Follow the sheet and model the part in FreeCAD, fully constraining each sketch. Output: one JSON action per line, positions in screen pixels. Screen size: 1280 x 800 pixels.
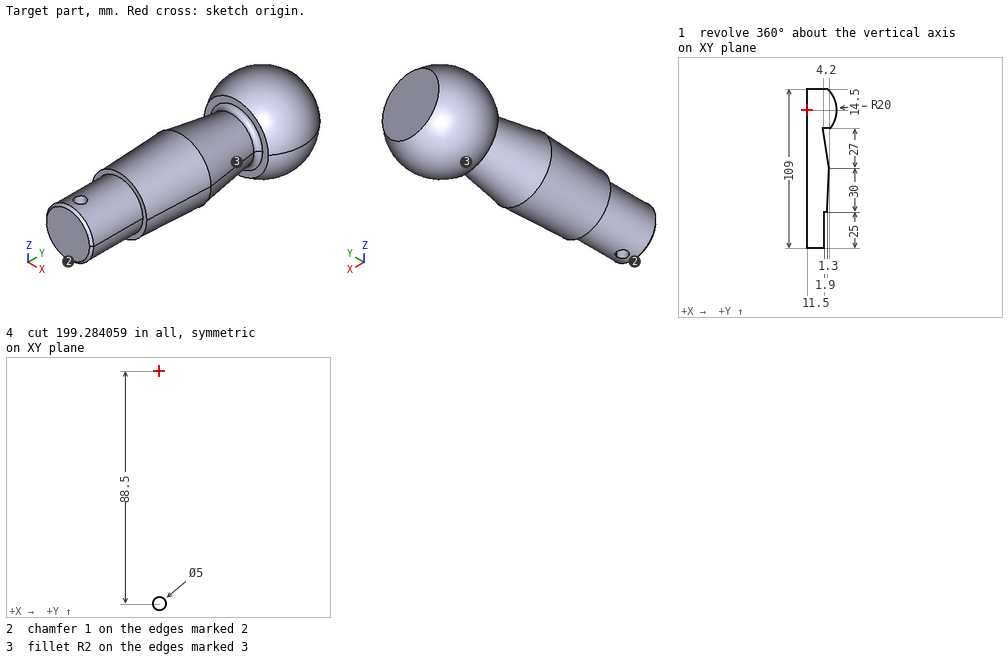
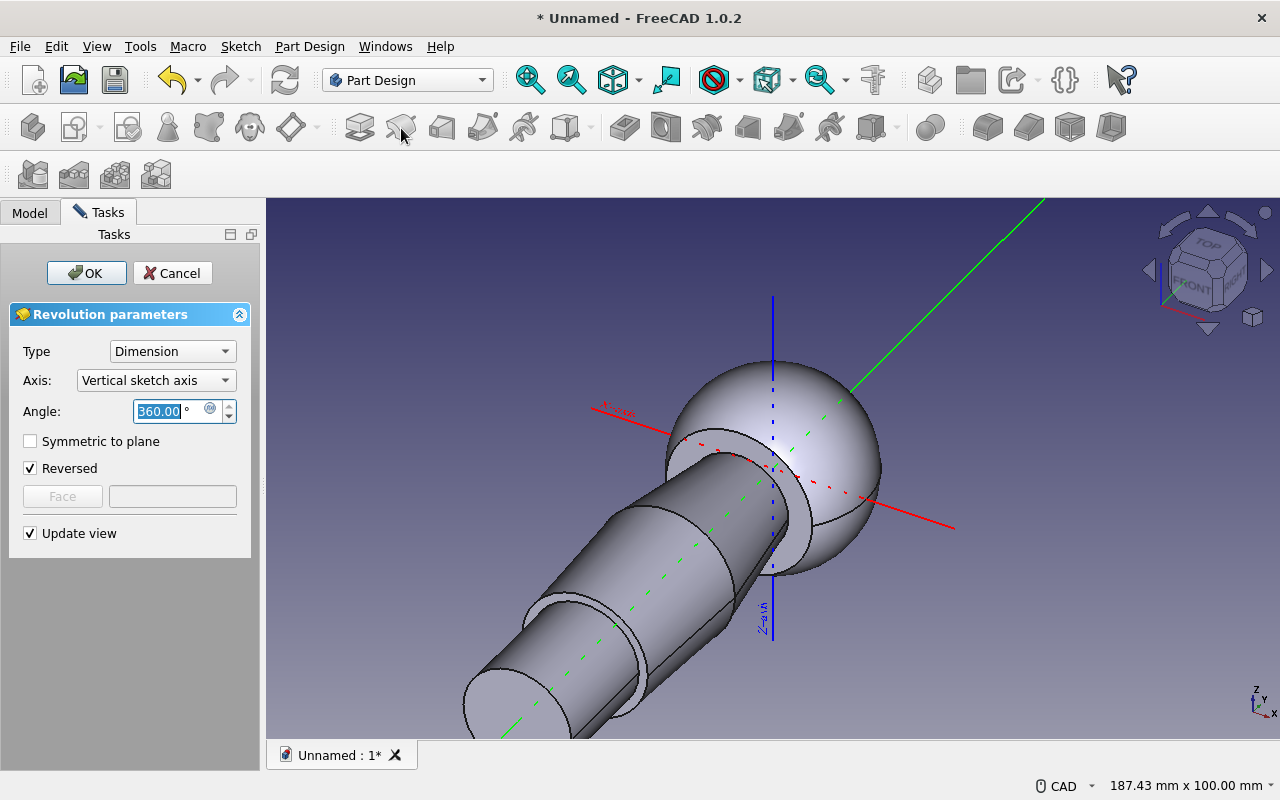
{"action": "left_click", "coordinate": [87, 273]}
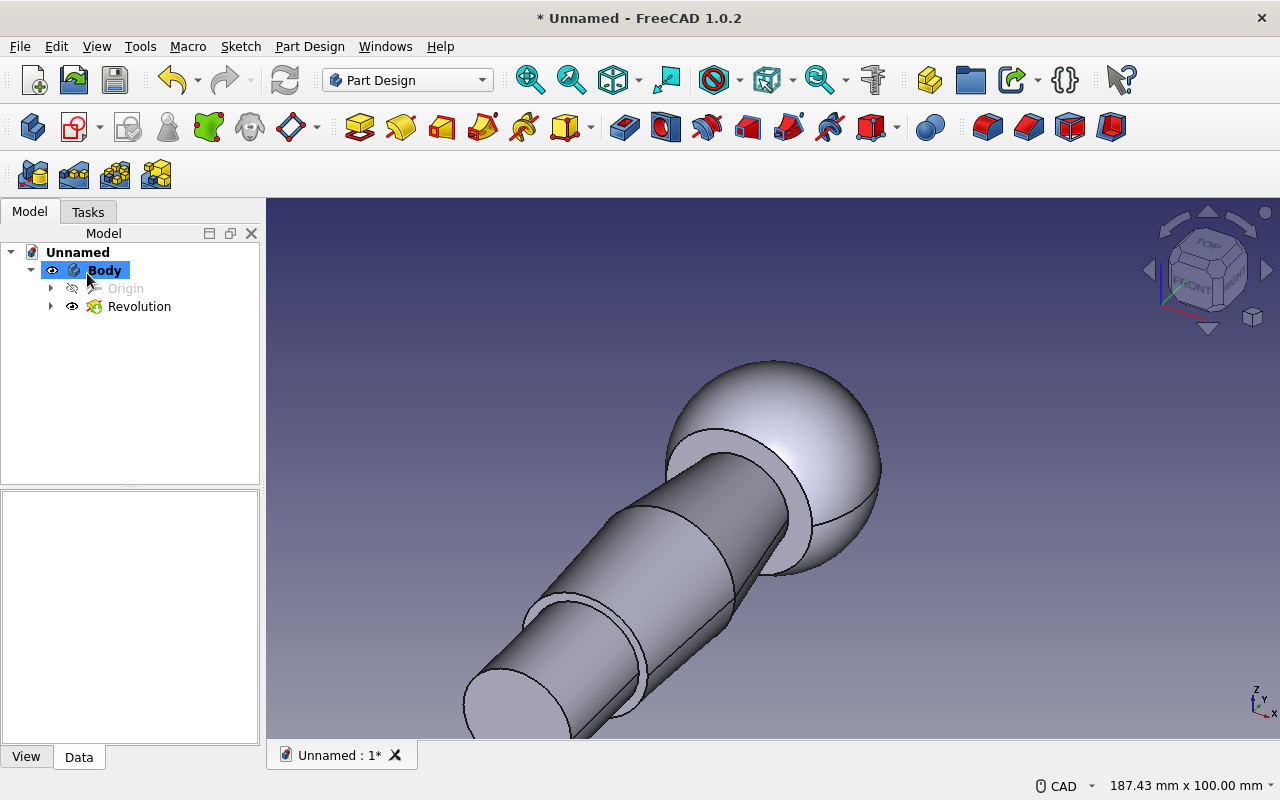
{"action": "left_click", "coordinate": [531, 80]}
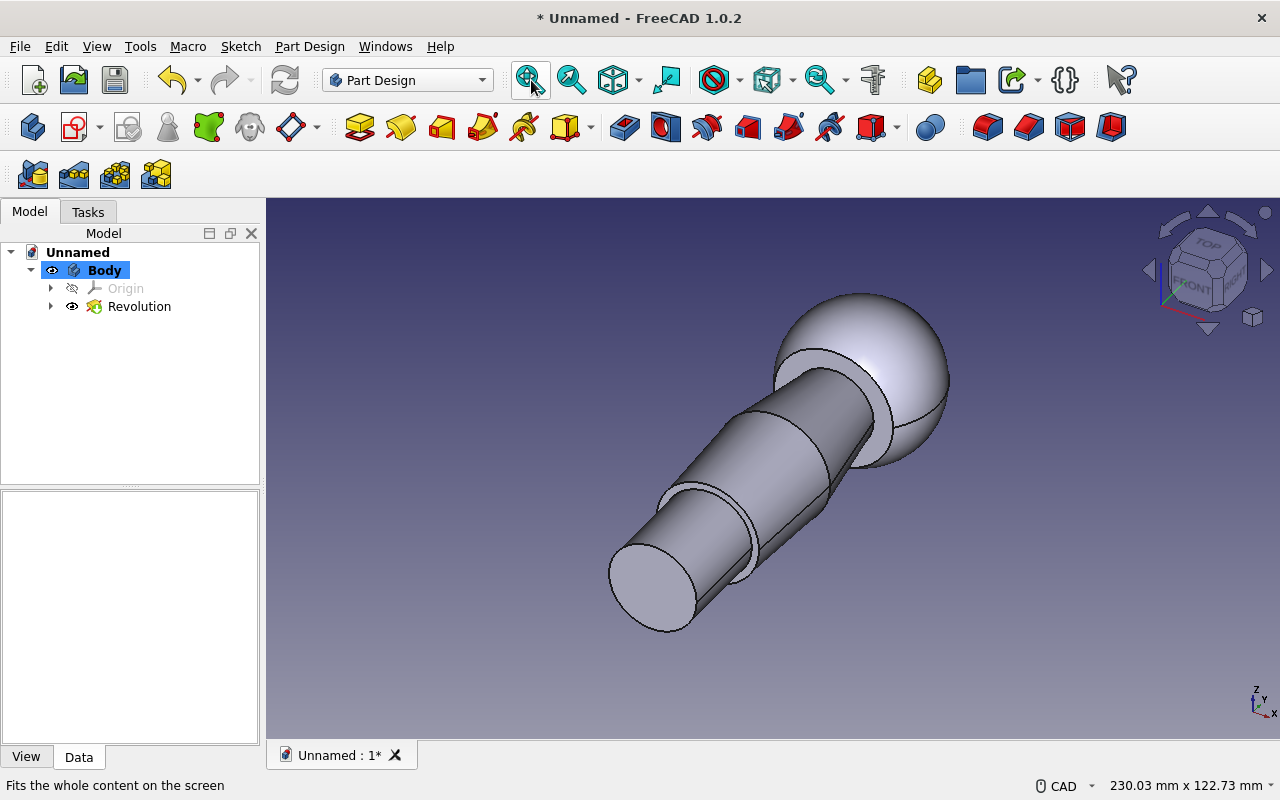
{"action": "left_click", "coordinate": [617, 551]}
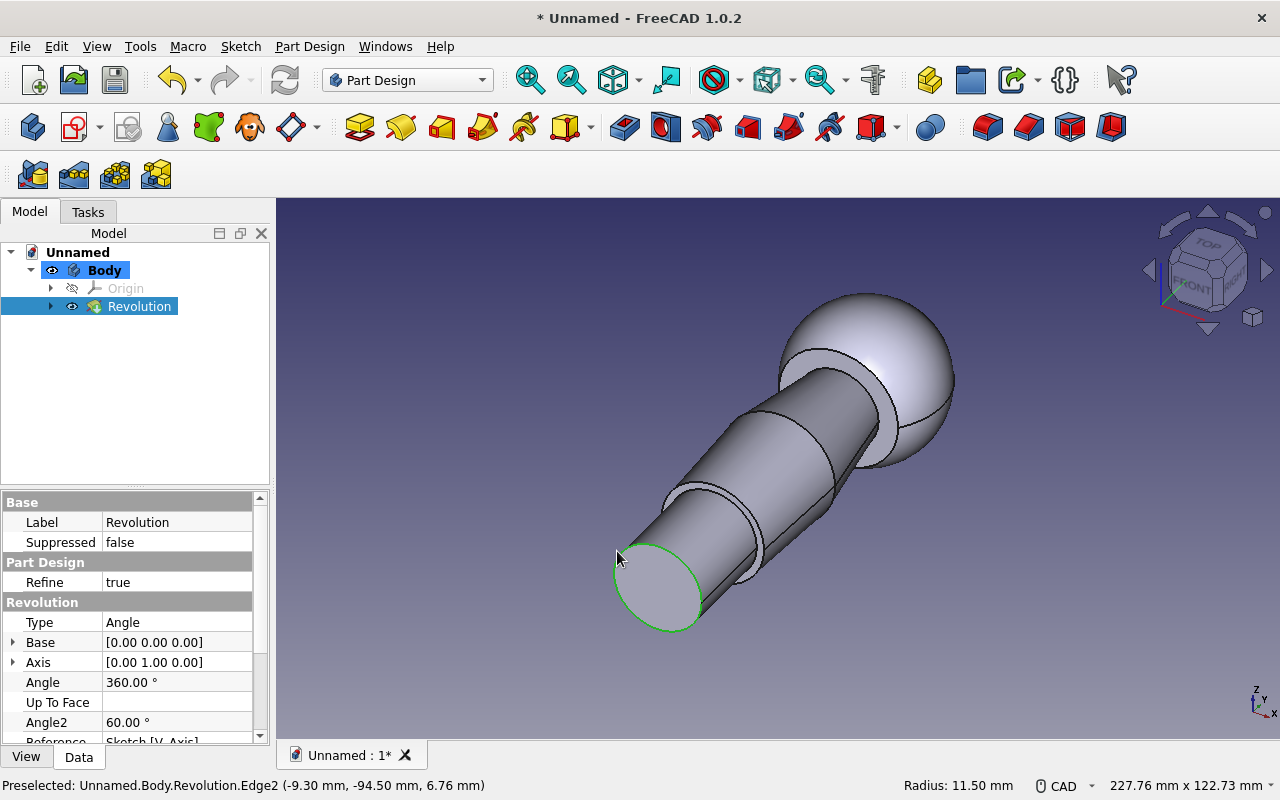
{"action": "left_click", "coordinate": [1029, 128]}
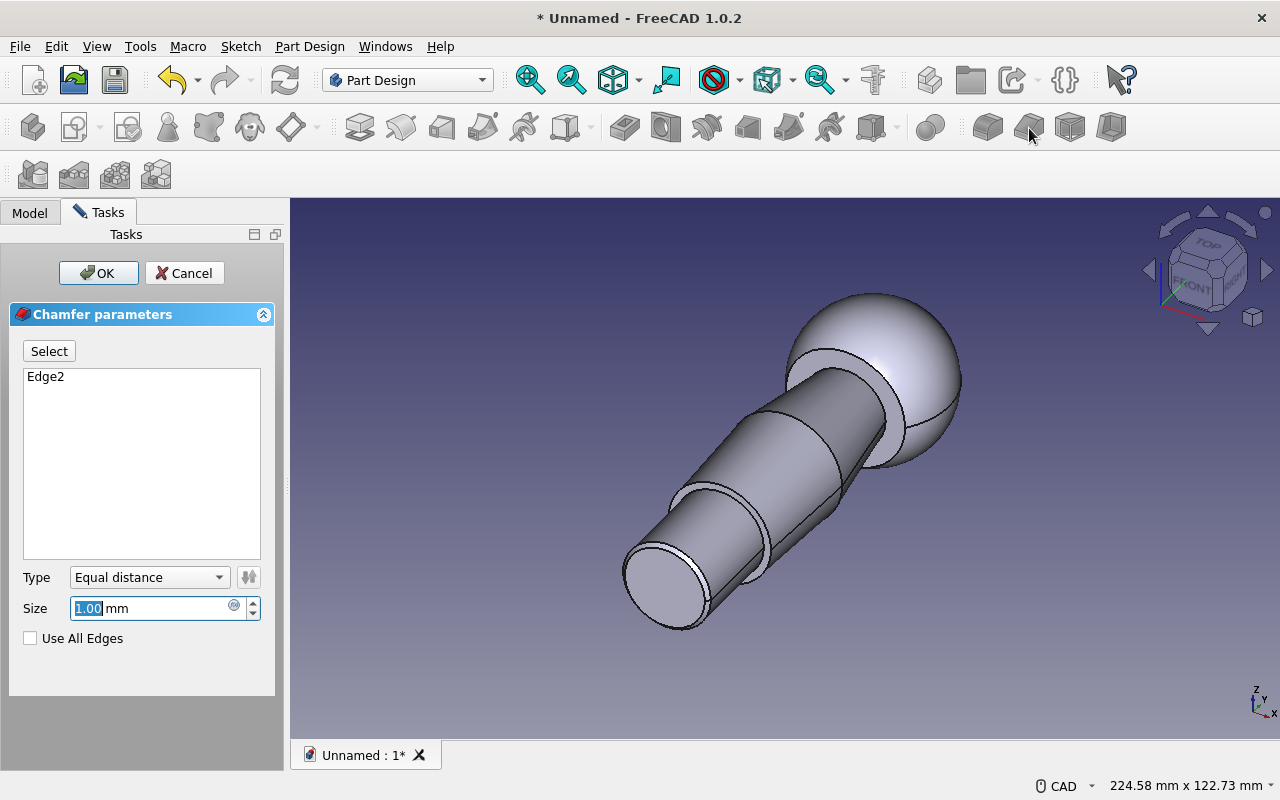
{"action": "type", "text": "1"}
{"action": "key", "text": "Tab"}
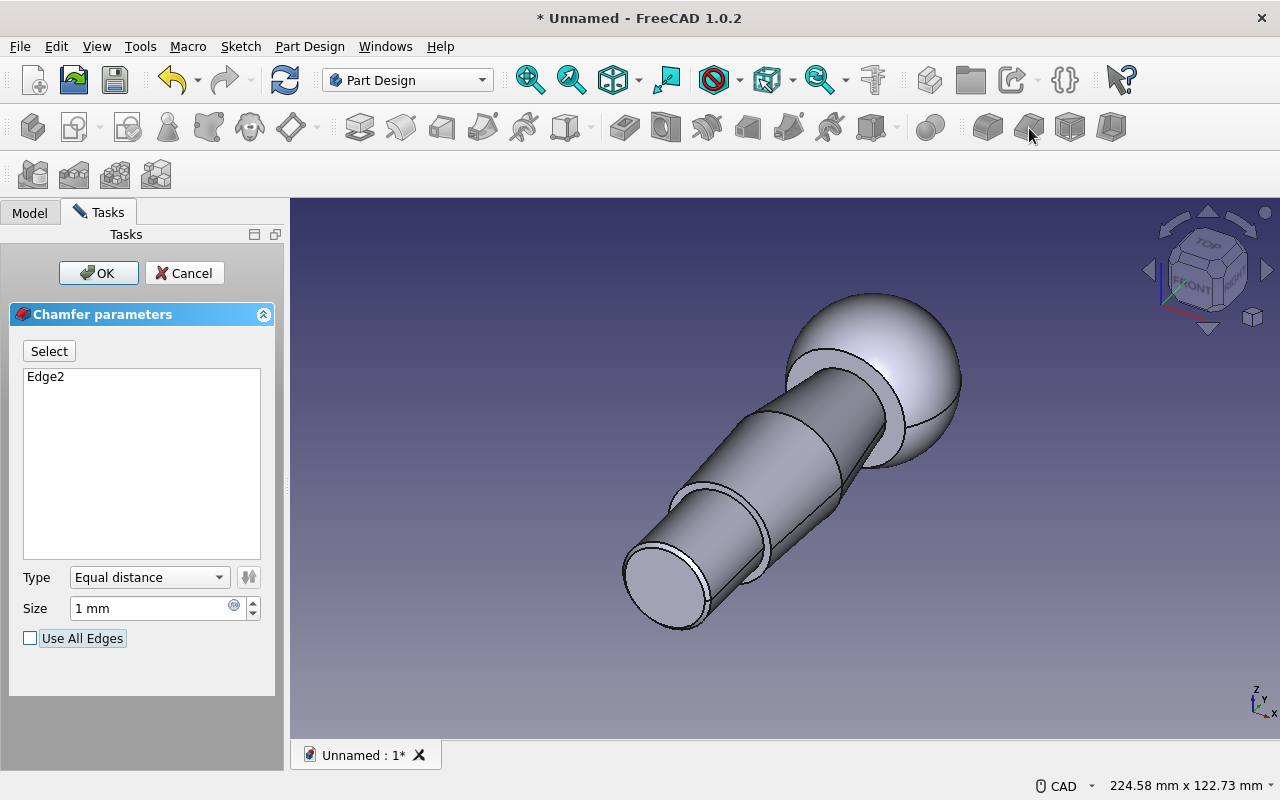
{"action": "left_click", "coordinate": [99, 273]}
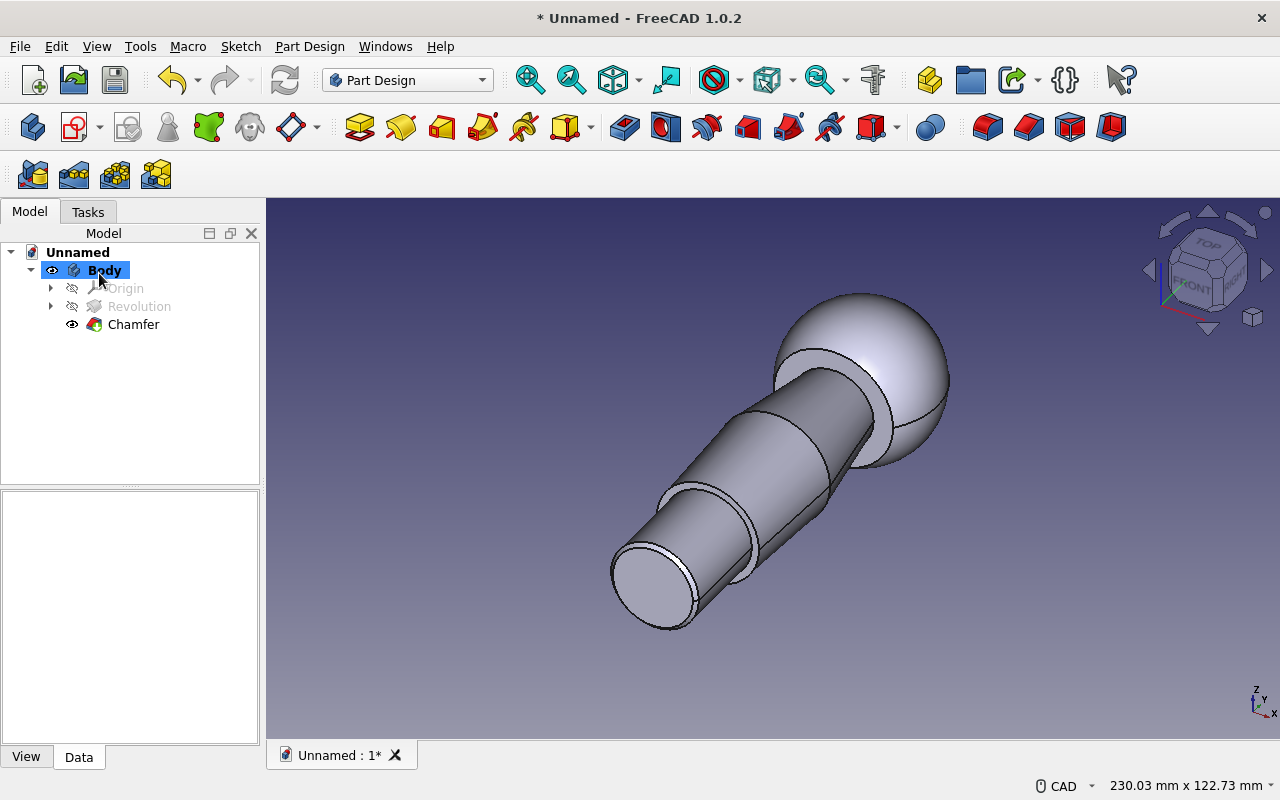
{"action": "key", "text": "0"}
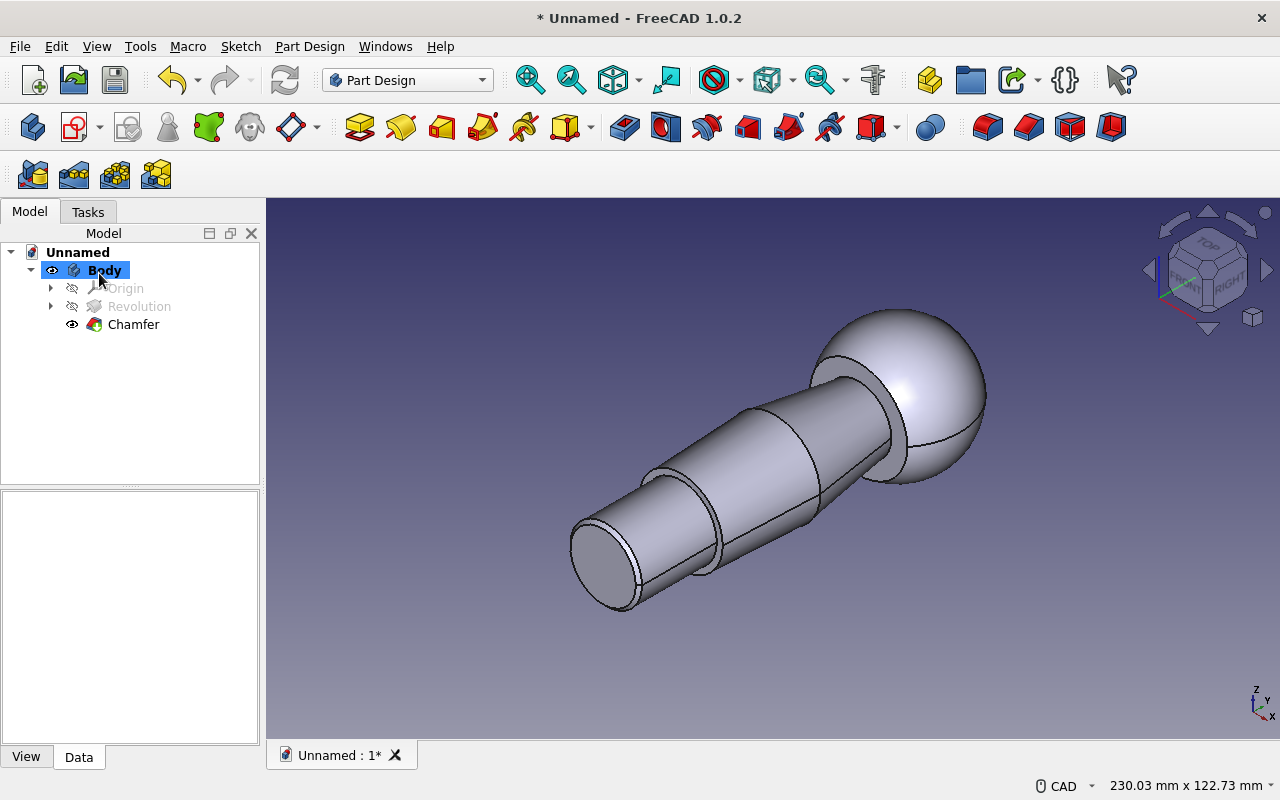
{"action": "key", "text": "2"}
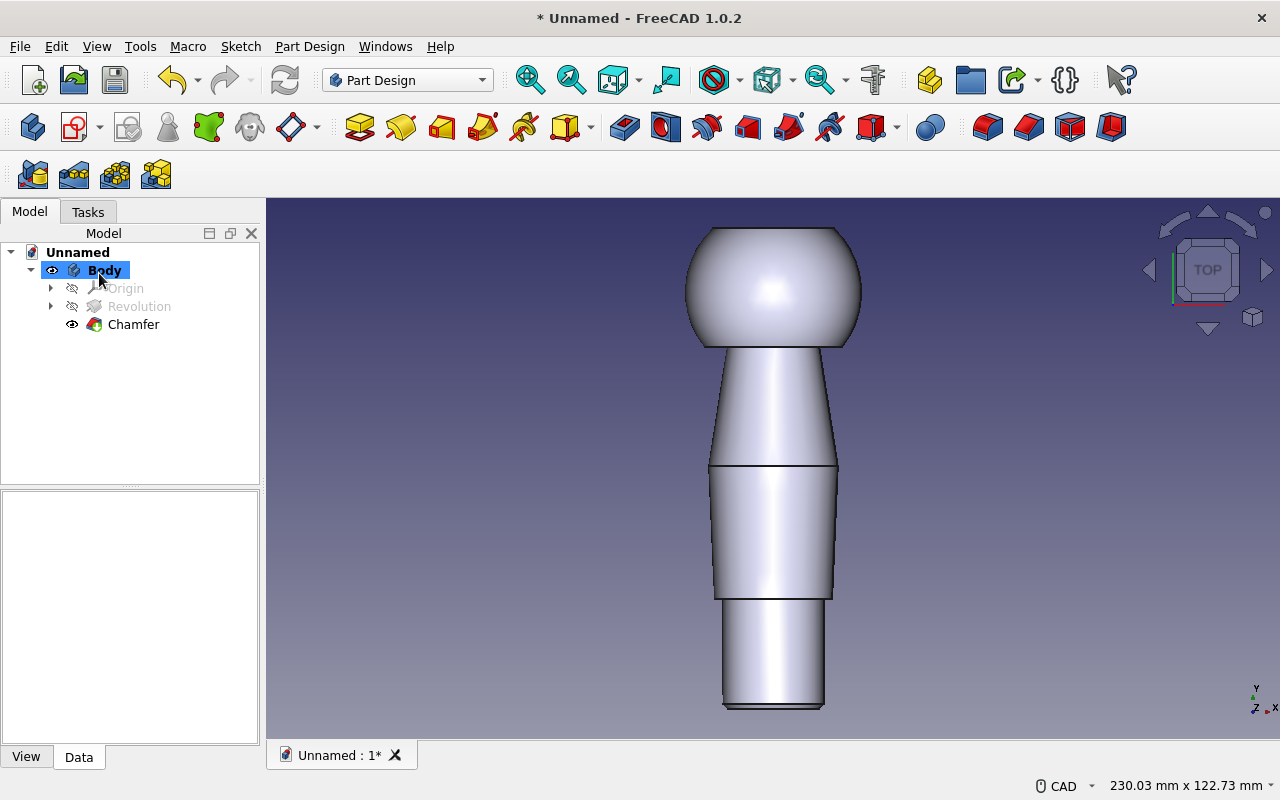
{"action": "key", "text": "1"}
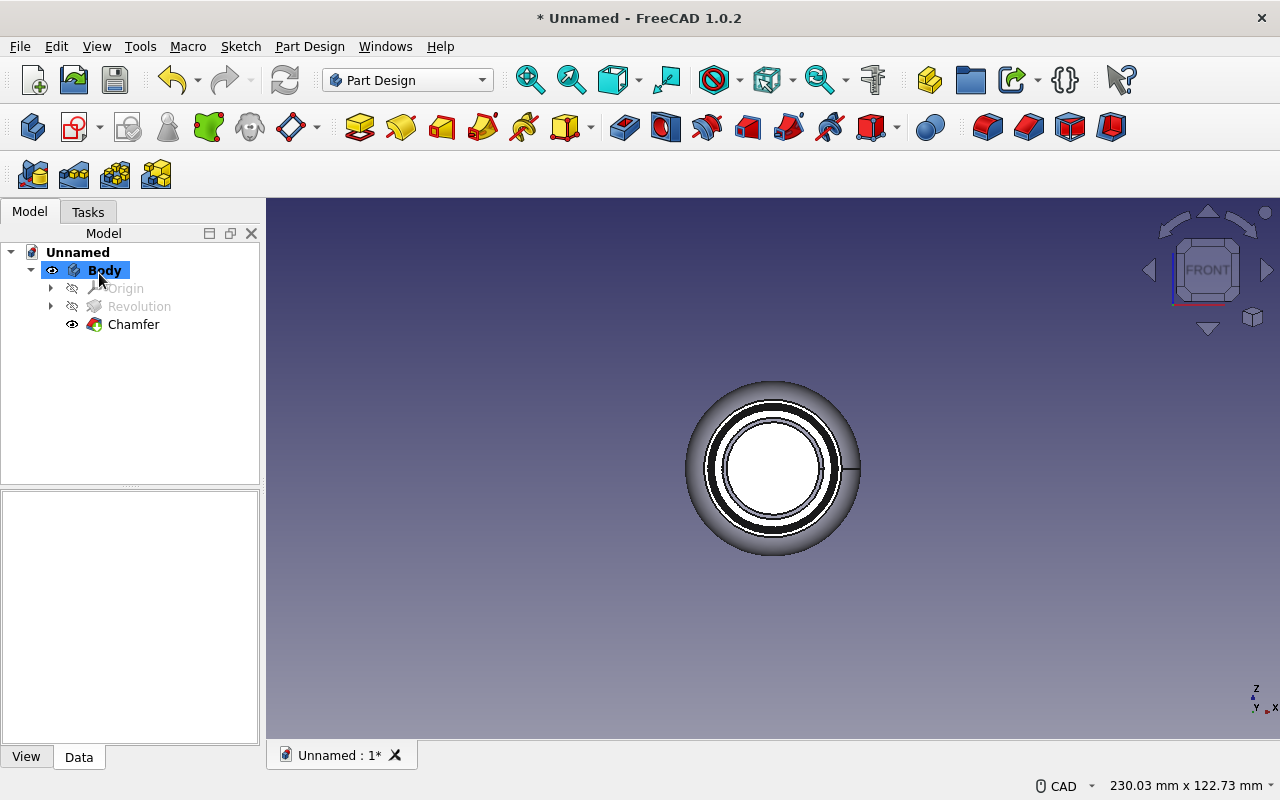
{"action": "left_click", "coordinate": [531, 80]}